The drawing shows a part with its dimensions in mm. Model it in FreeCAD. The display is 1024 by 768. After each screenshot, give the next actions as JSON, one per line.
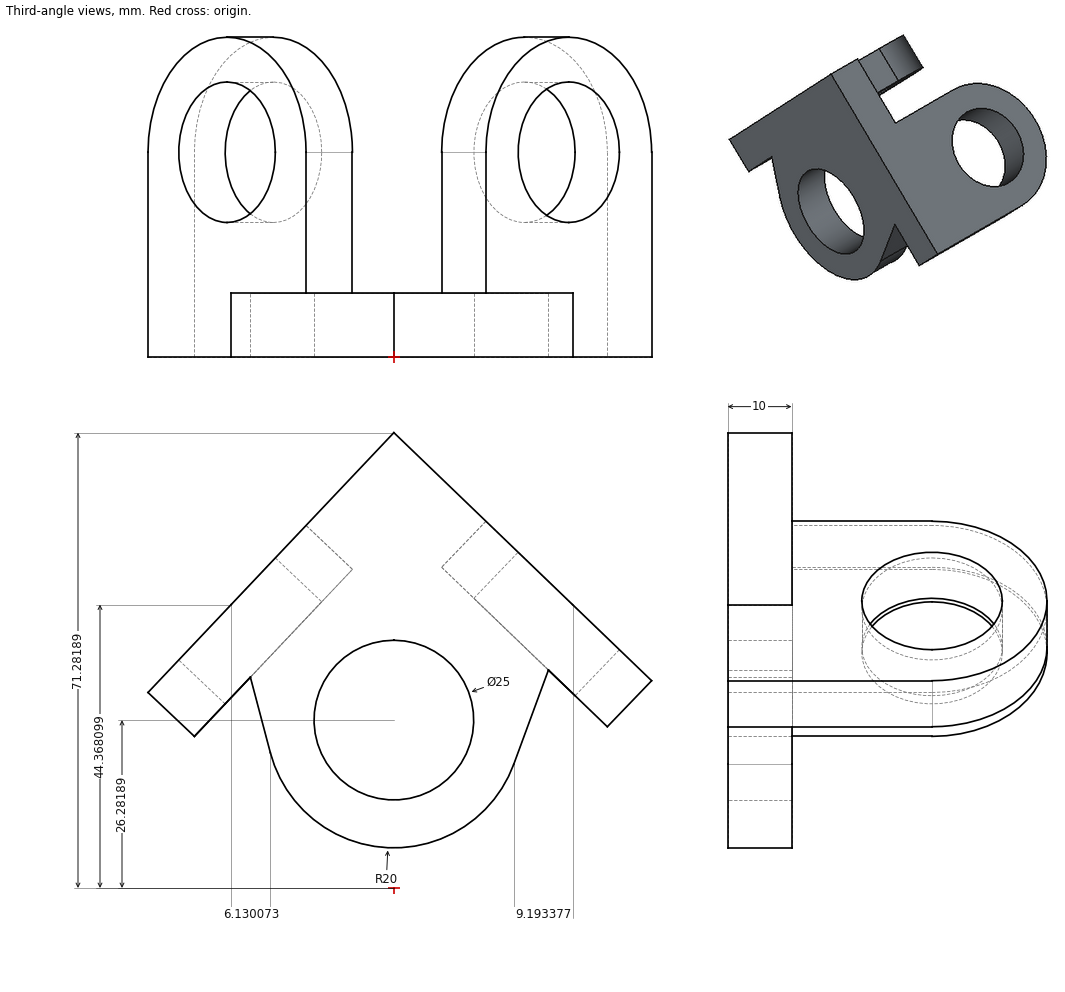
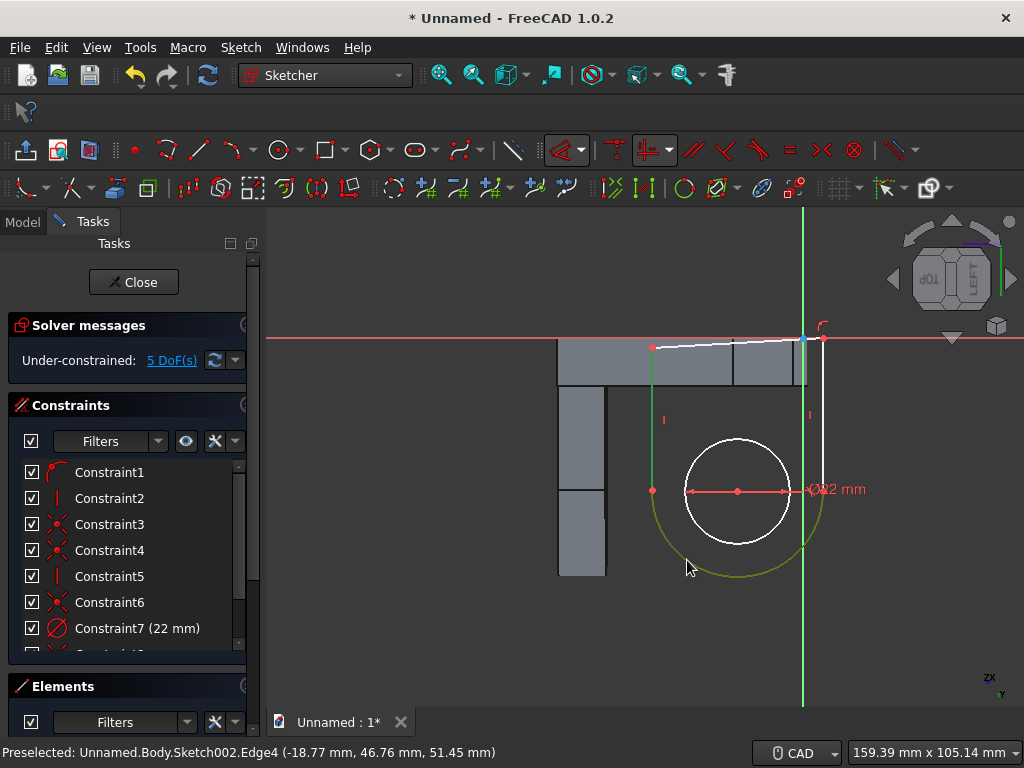
{"action": "left_click", "coordinate": [758, 150]}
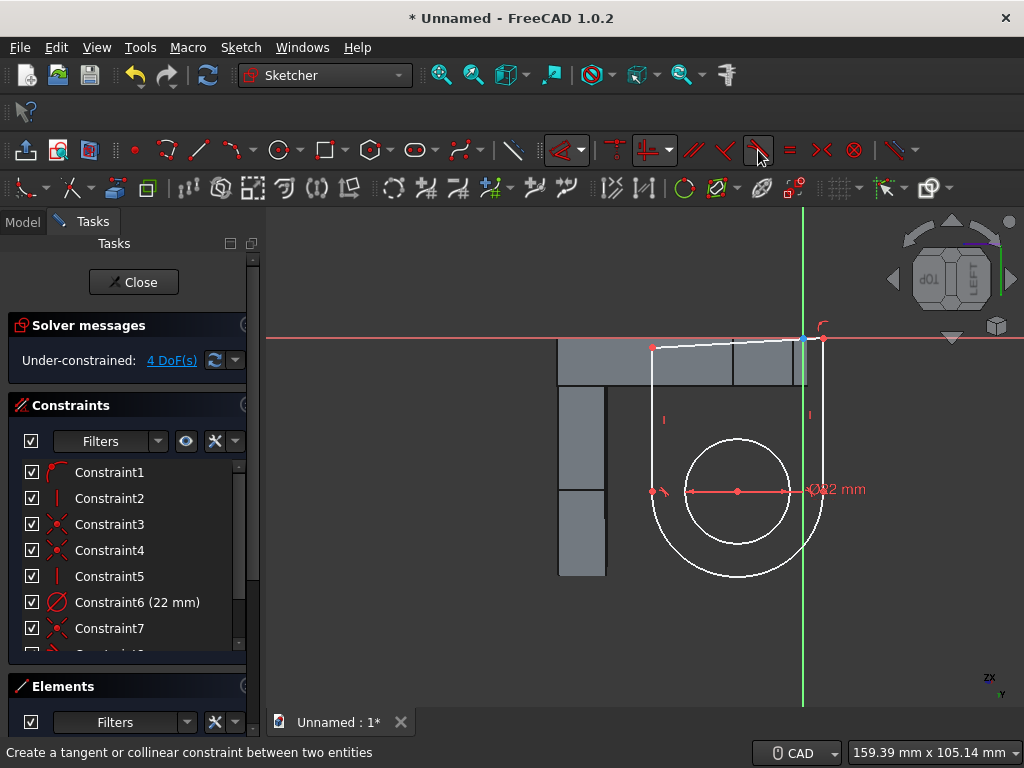
{"action": "left_click", "coordinate": [772, 341]}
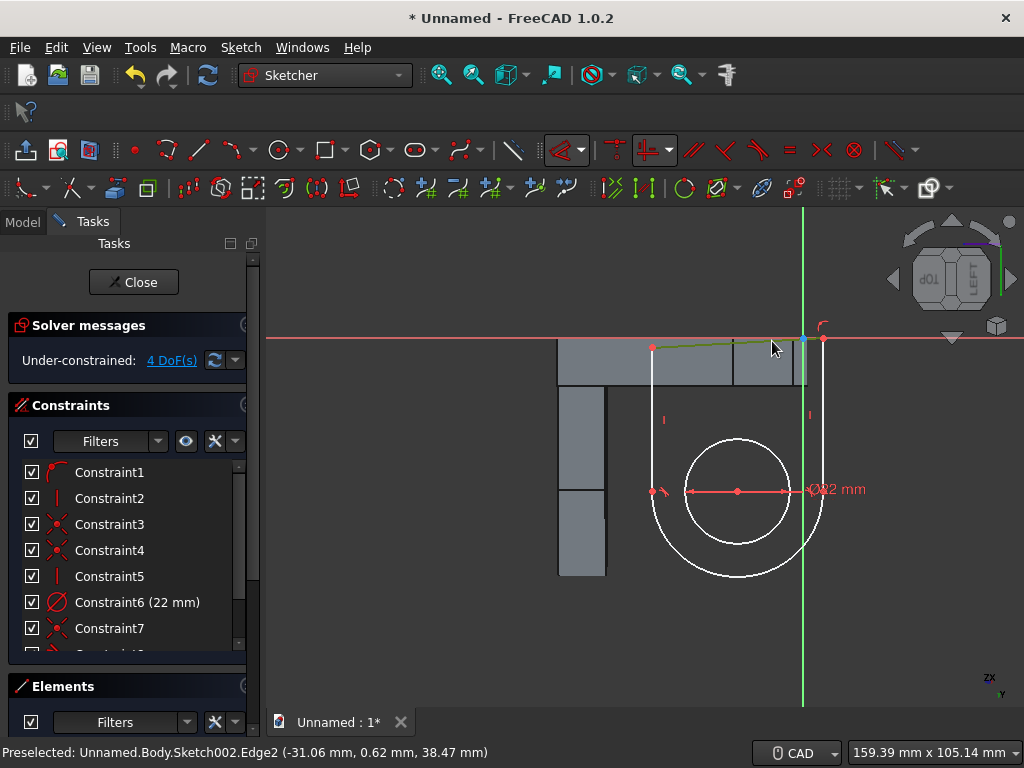
{"action": "left_click", "coordinate": [672, 150]}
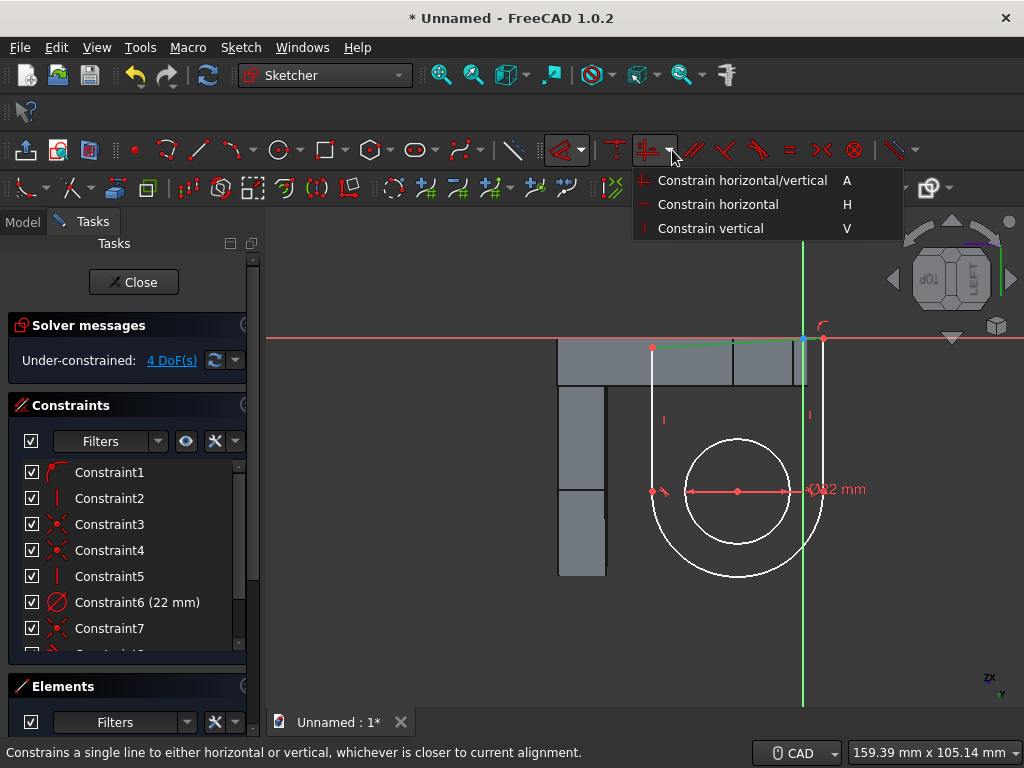
{"action": "left_click", "coordinate": [768, 204]}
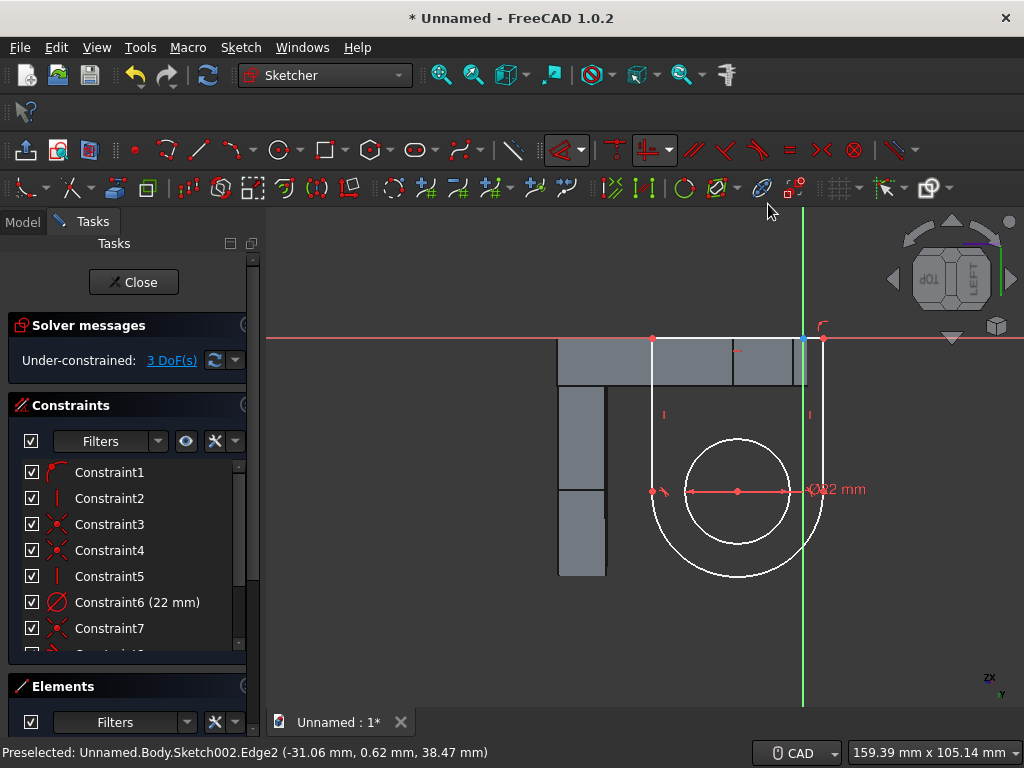
{"action": "left_click", "coordinate": [687, 561]}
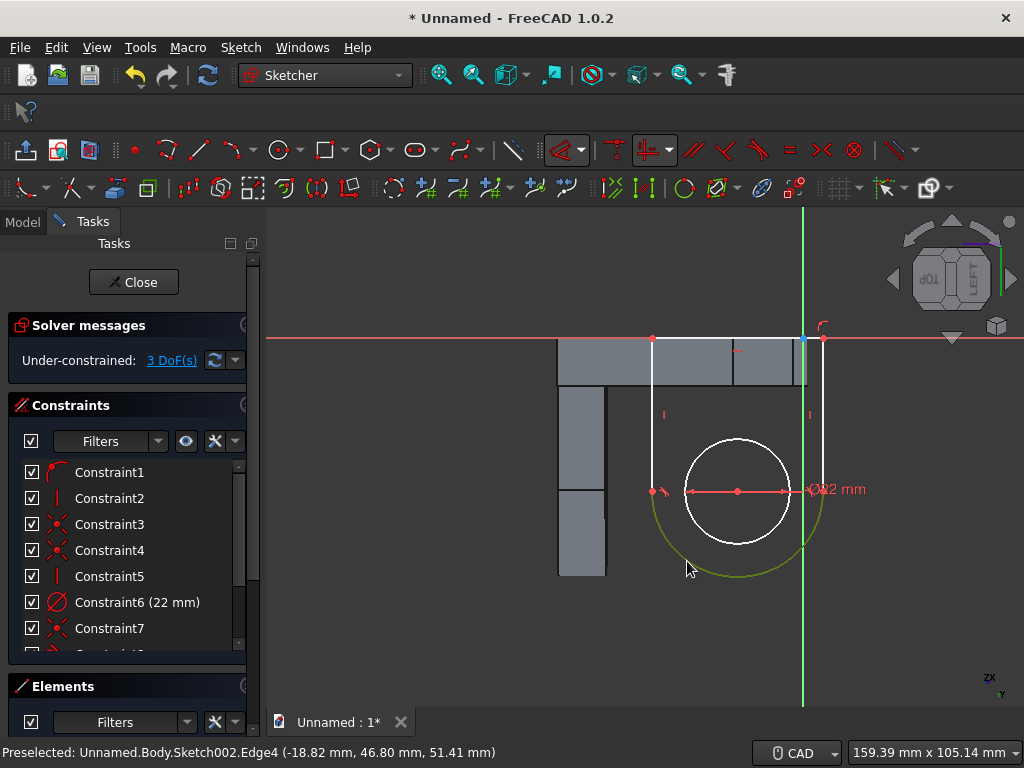
{"action": "left_click", "coordinate": [584, 150]}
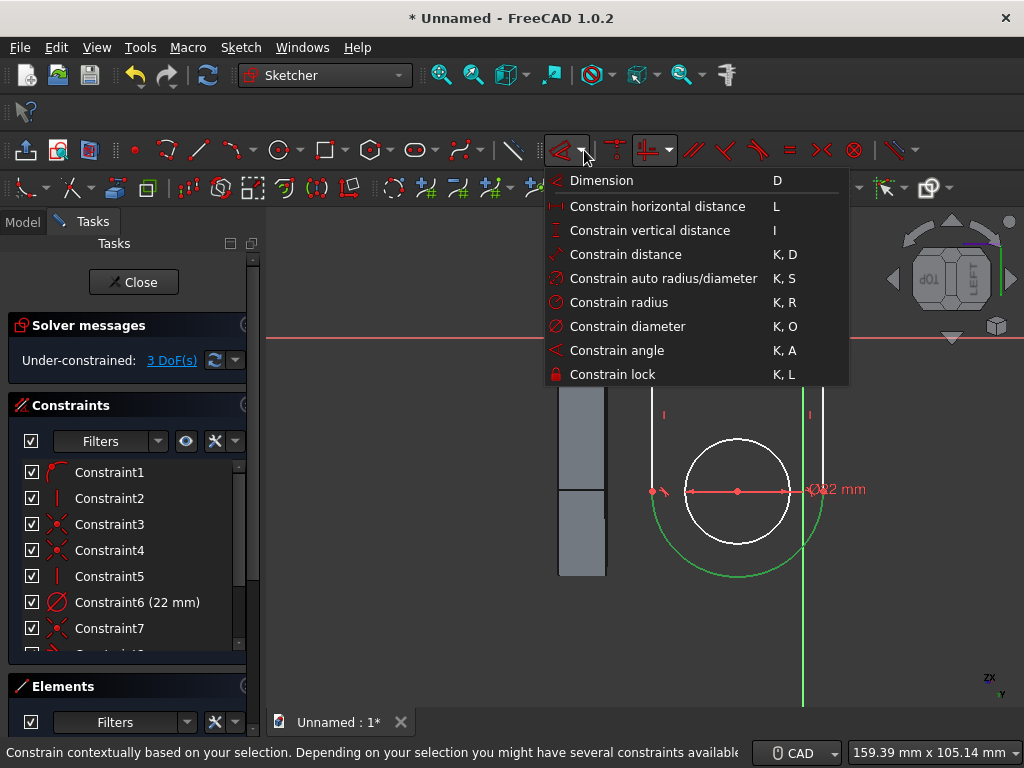
{"action": "left_click", "coordinate": [697, 302]}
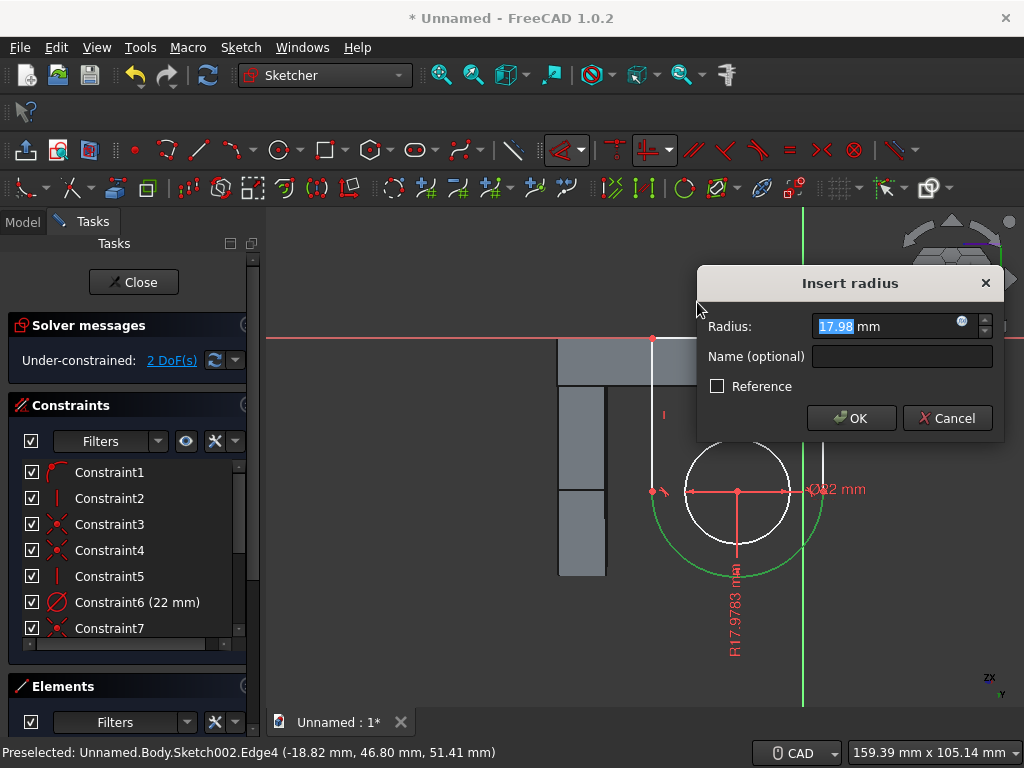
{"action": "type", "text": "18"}
{"action": "key", "text": "Return"}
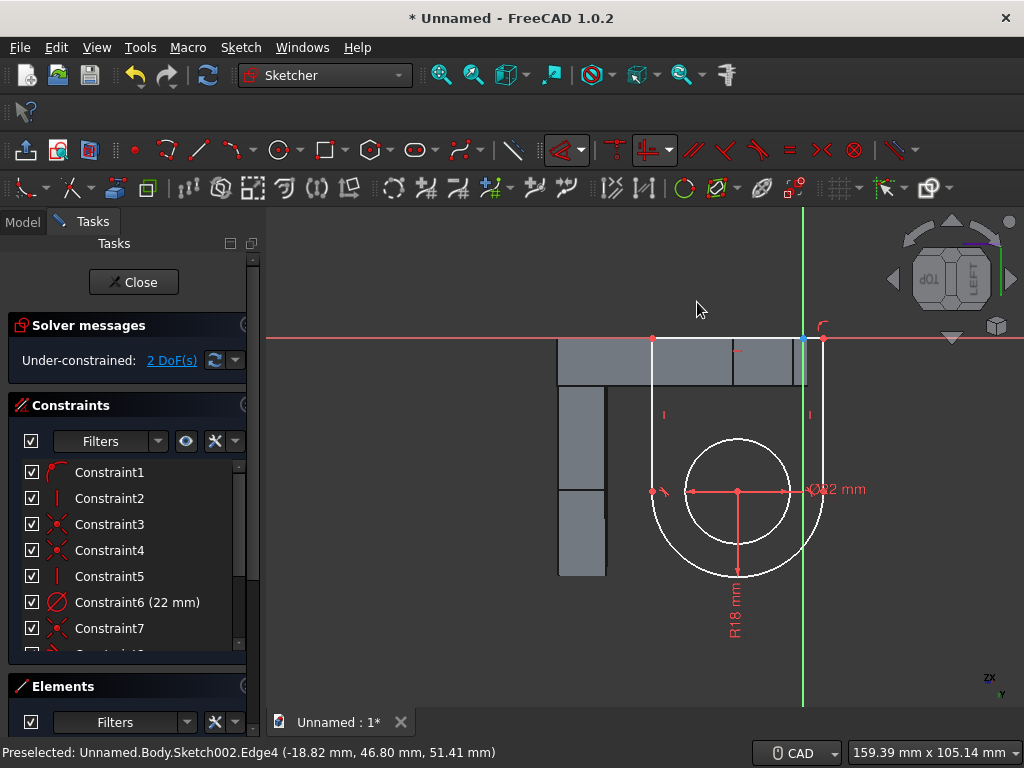
{"action": "left_click", "coordinate": [823, 445]}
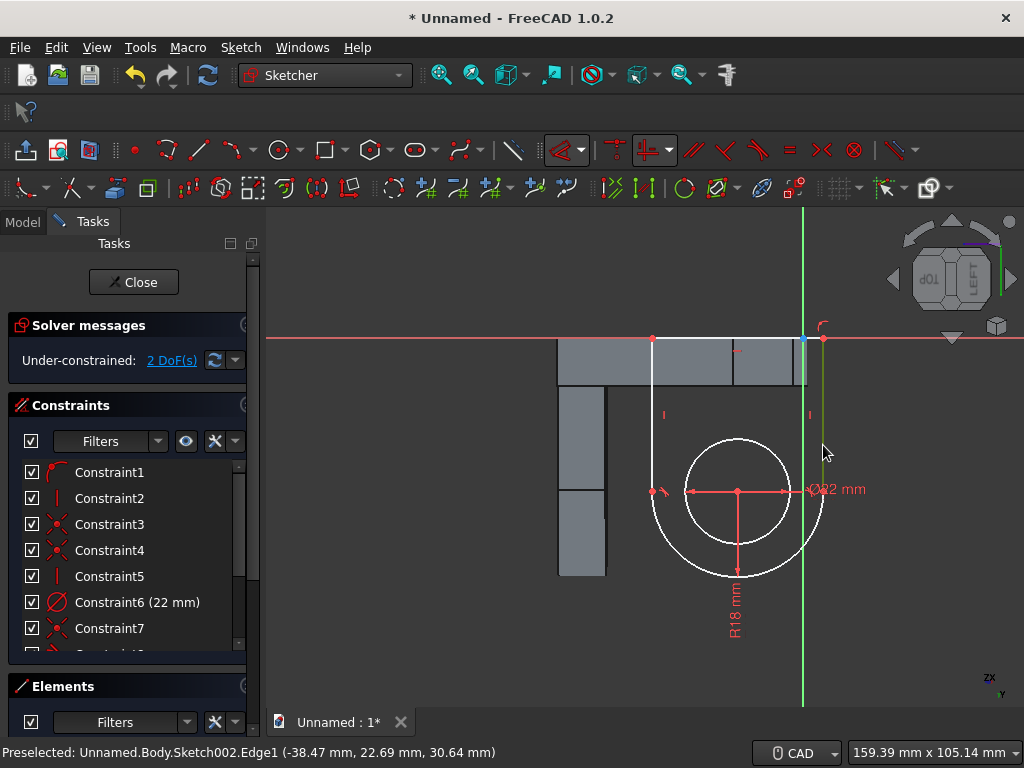
{"action": "left_click", "coordinate": [584, 150]}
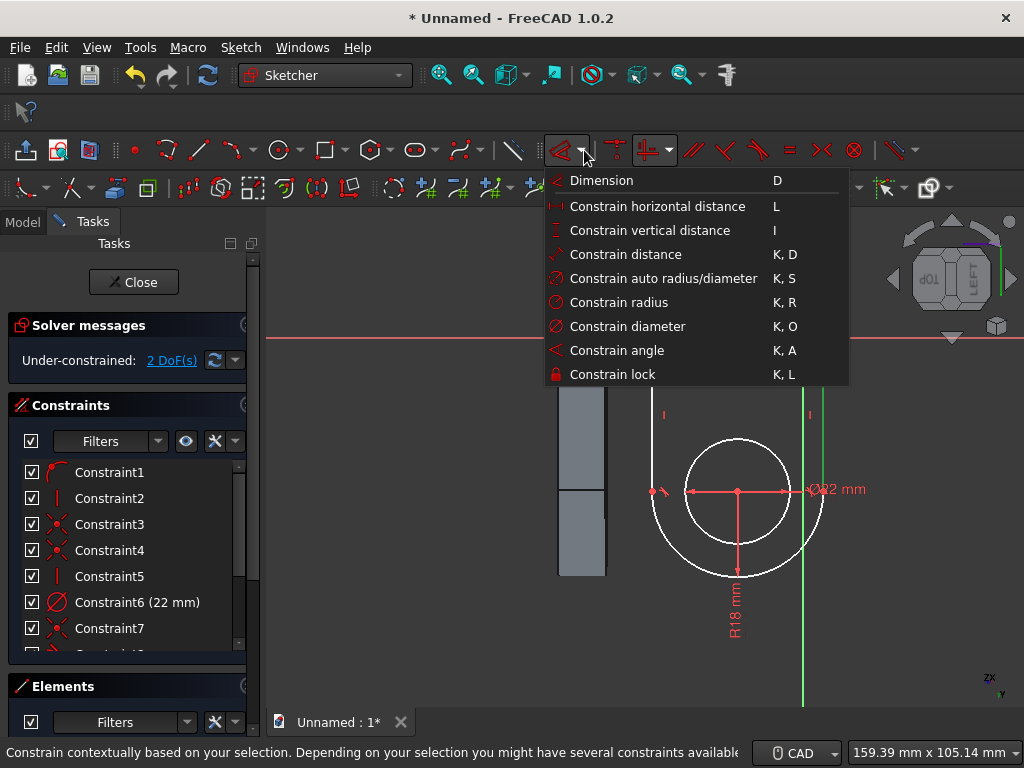
{"action": "left_click", "coordinate": [697, 230]}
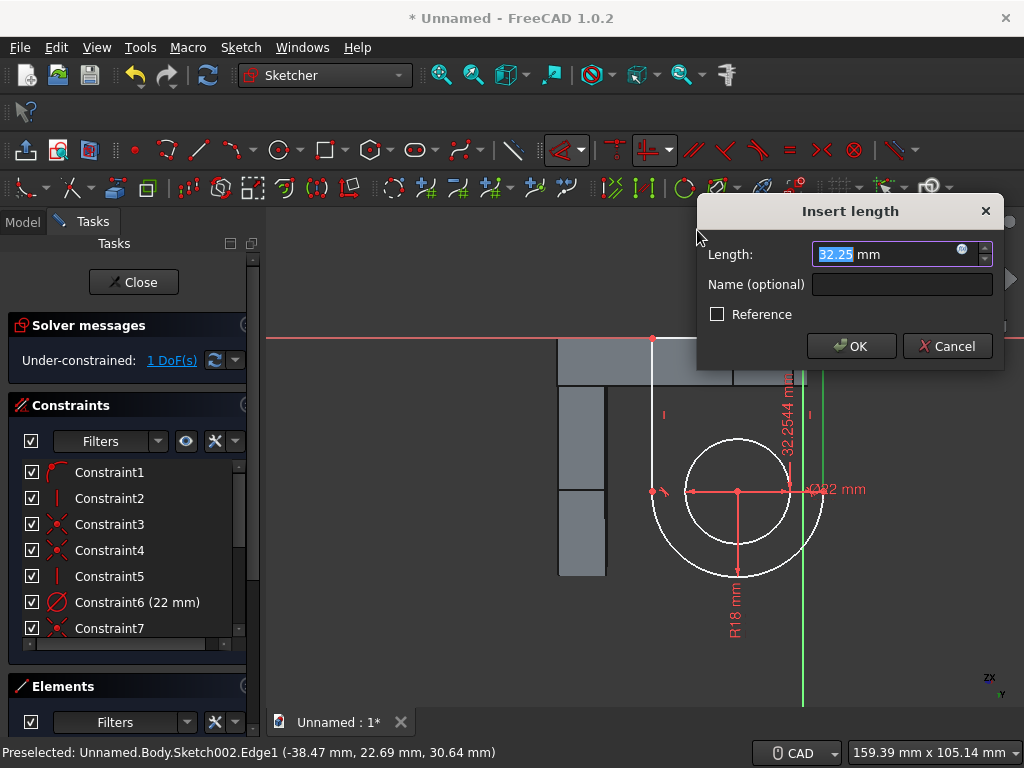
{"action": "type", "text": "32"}
{"action": "key", "text": "Return"}